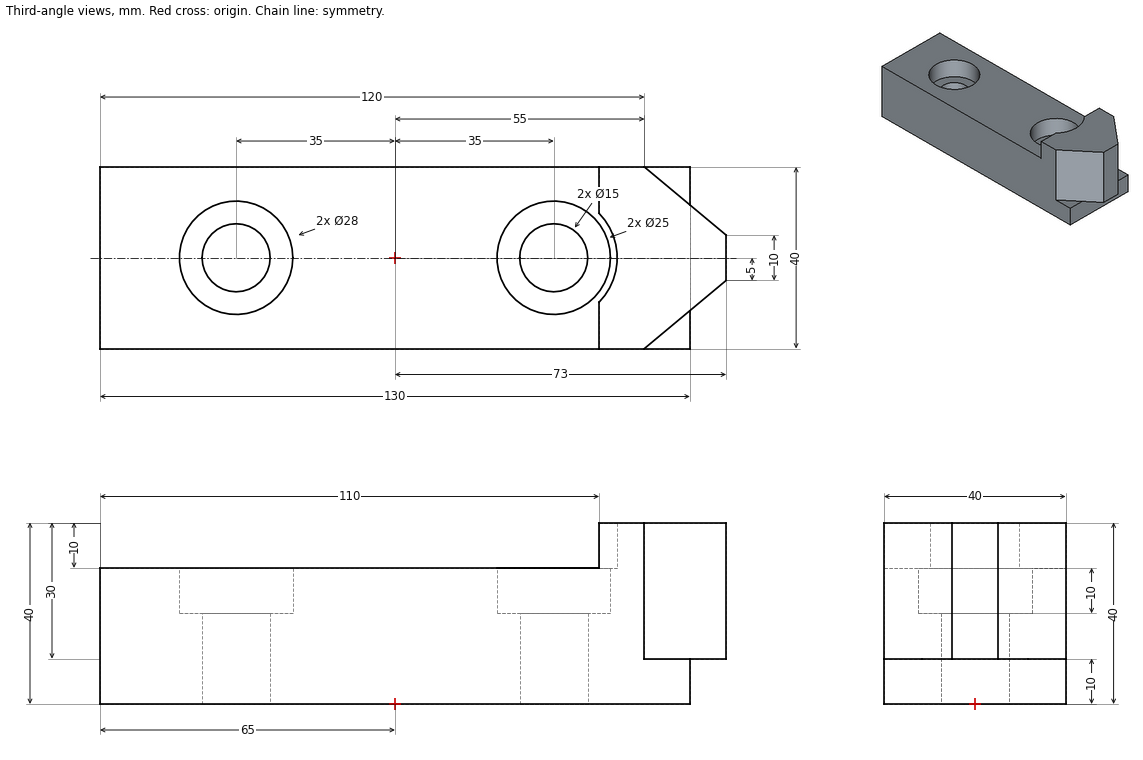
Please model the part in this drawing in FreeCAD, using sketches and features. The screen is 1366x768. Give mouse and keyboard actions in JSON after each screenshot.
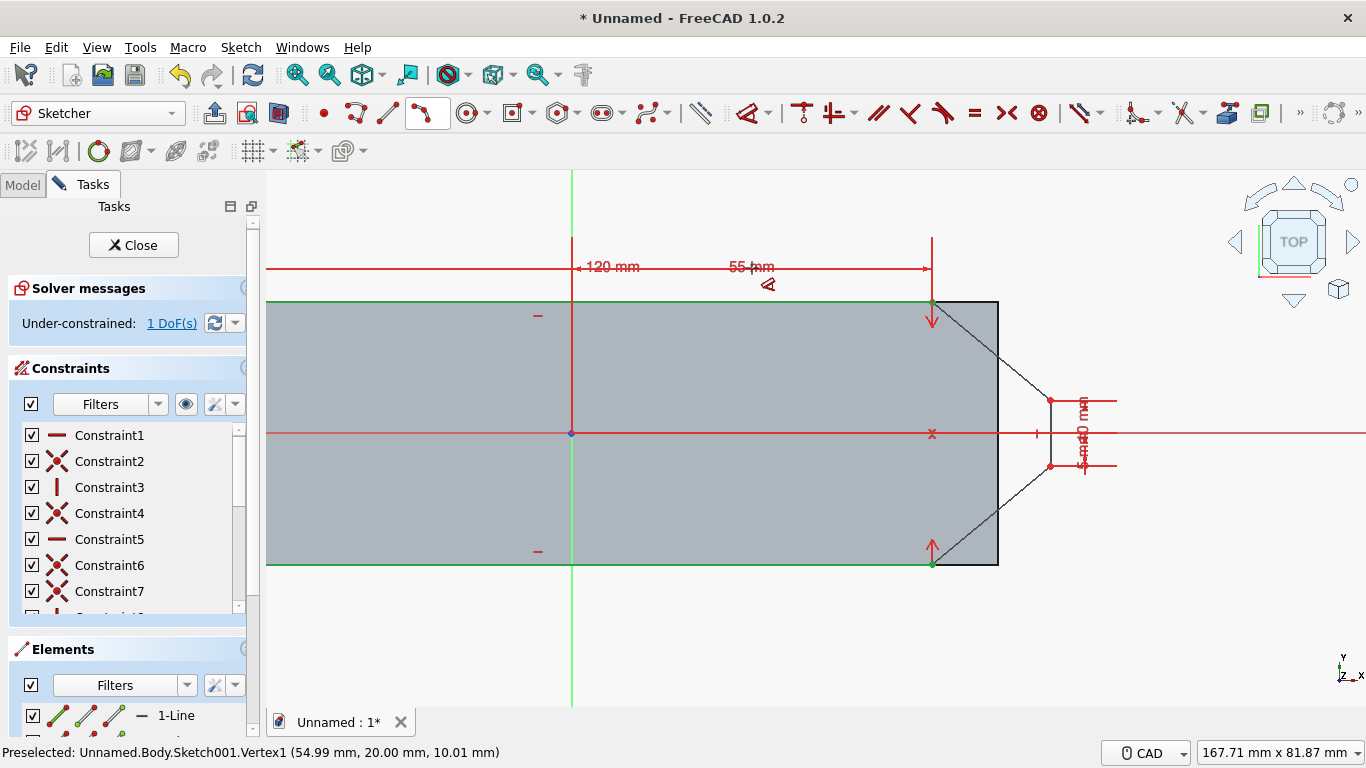
{"action": "left_click", "coordinate": [1051, 466]}
{"action": "left_click", "coordinate": [811, 500]}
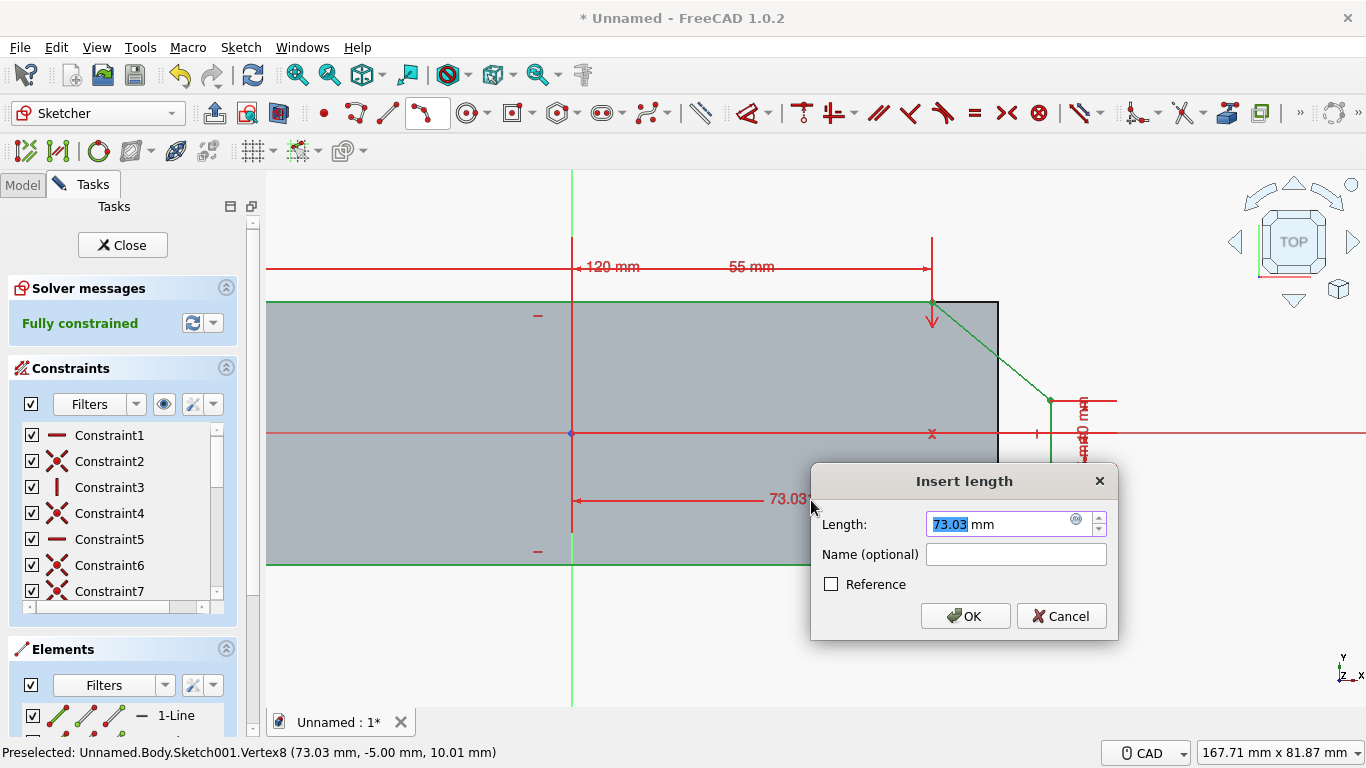
{"action": "type", "text": "73"}
{"action": "key", "text": "Return"}
{"action": "key", "text": "Escape"}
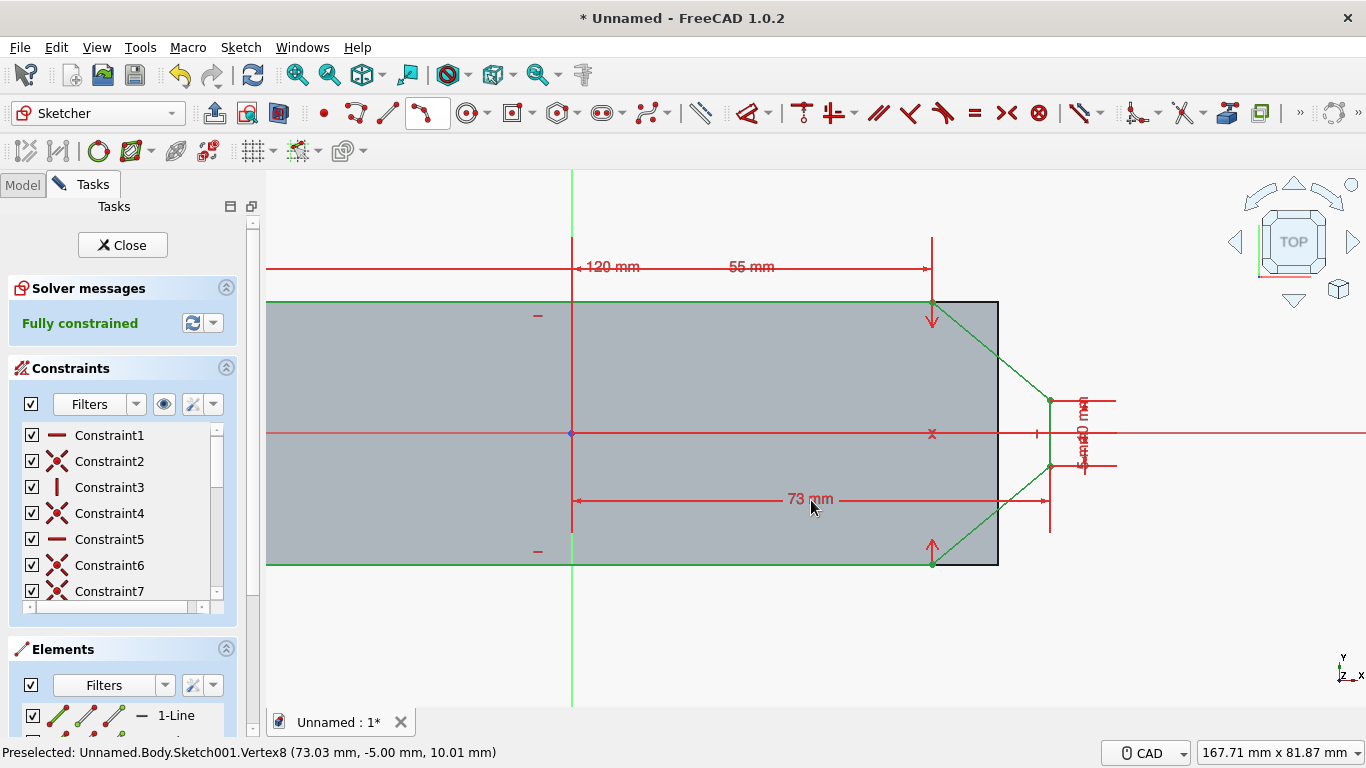
{"action": "left_click", "coordinate": [123, 245]}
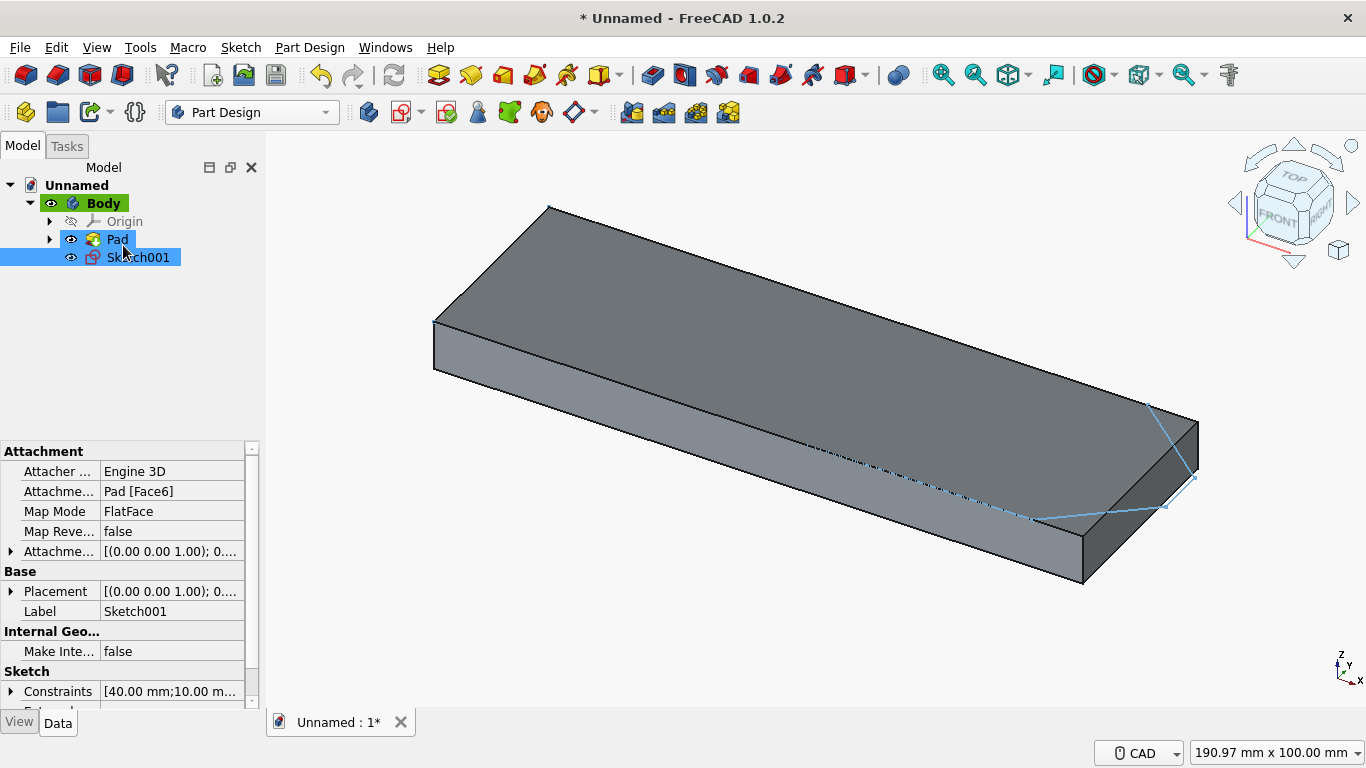
{"action": "left_click", "coordinate": [440, 76]}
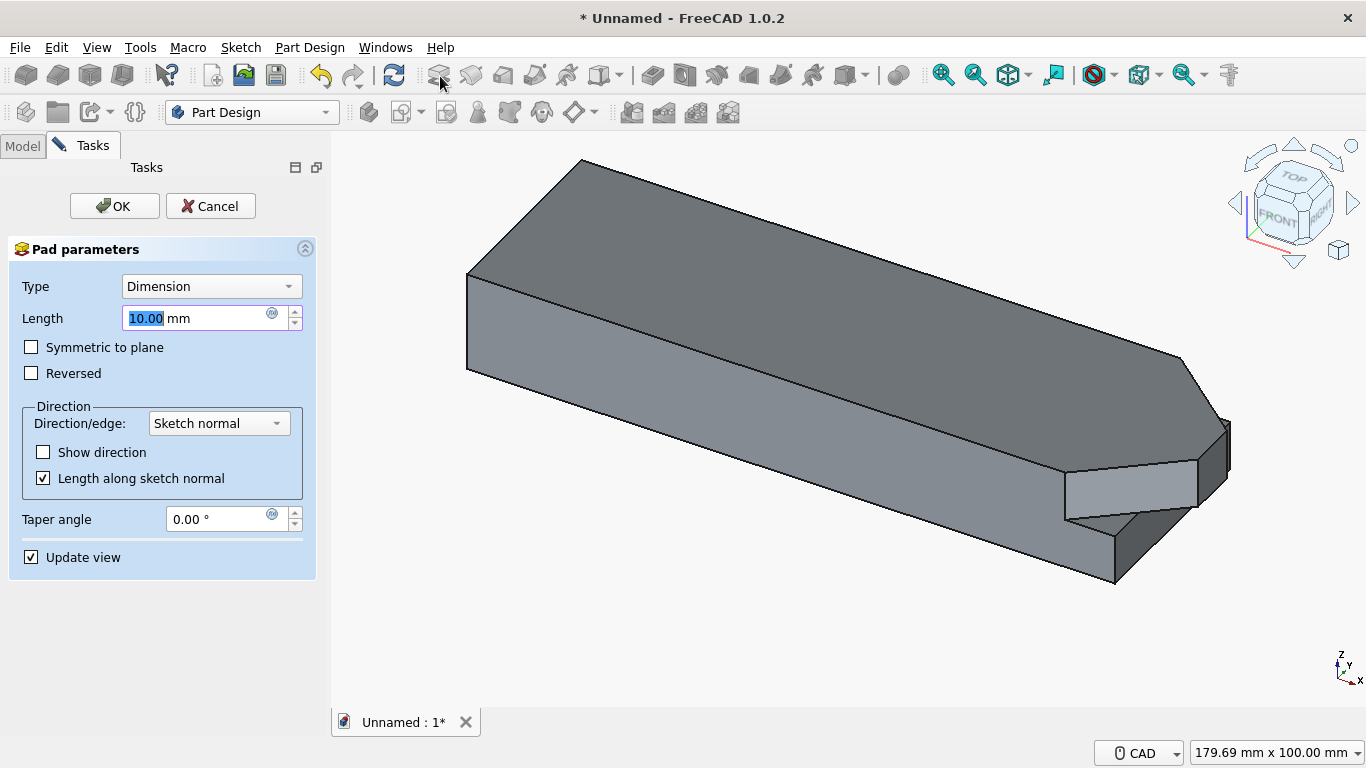
{"action": "type", "text": "30"}
{"action": "key", "text": "Tab"}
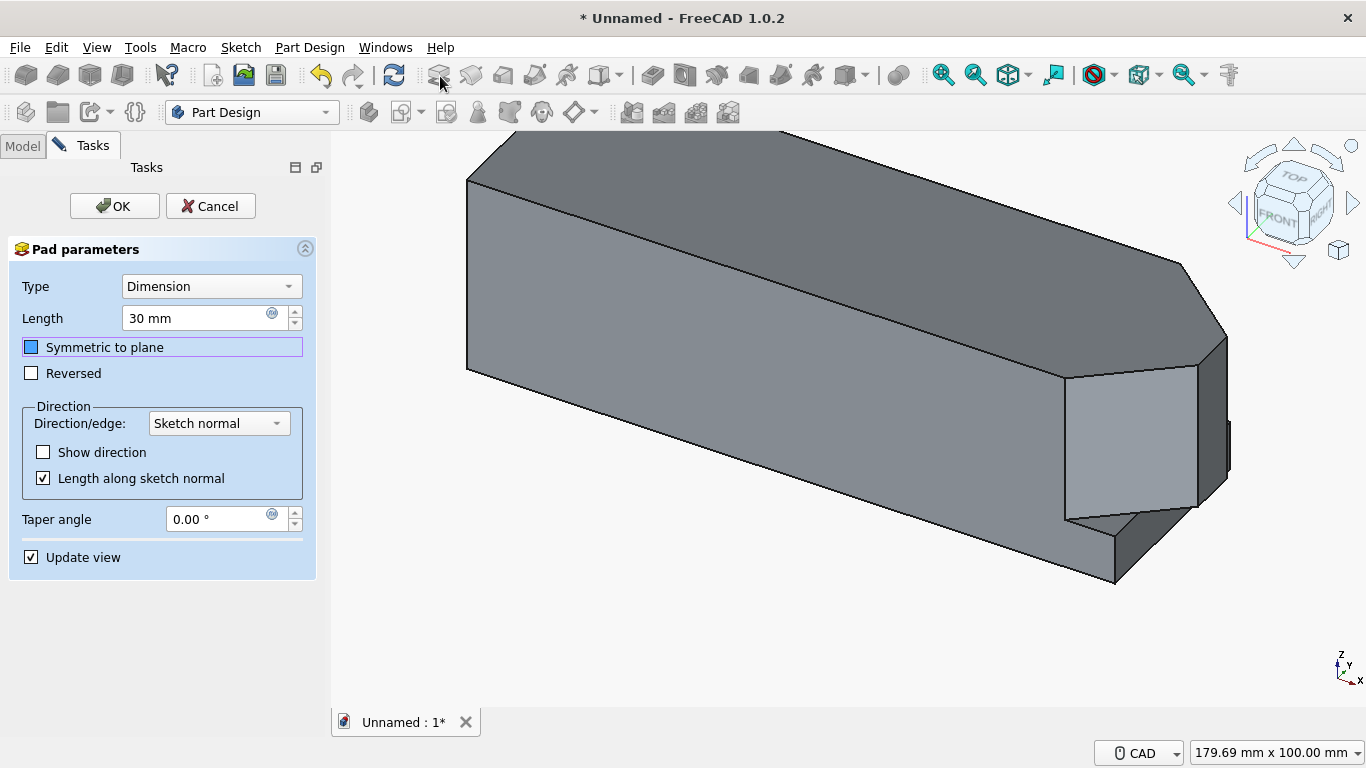
{"action": "left_click", "coordinate": [115, 206]}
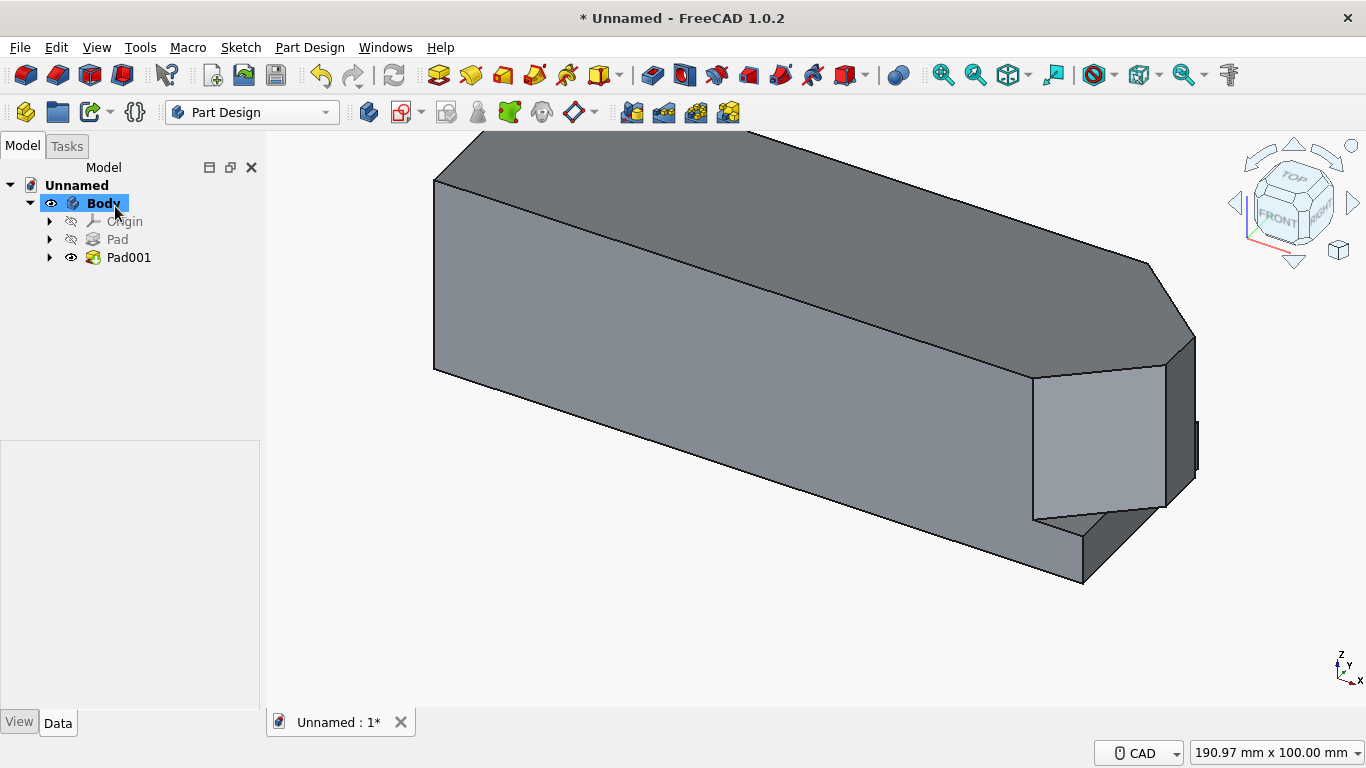
{"action": "key", "text": "v f"}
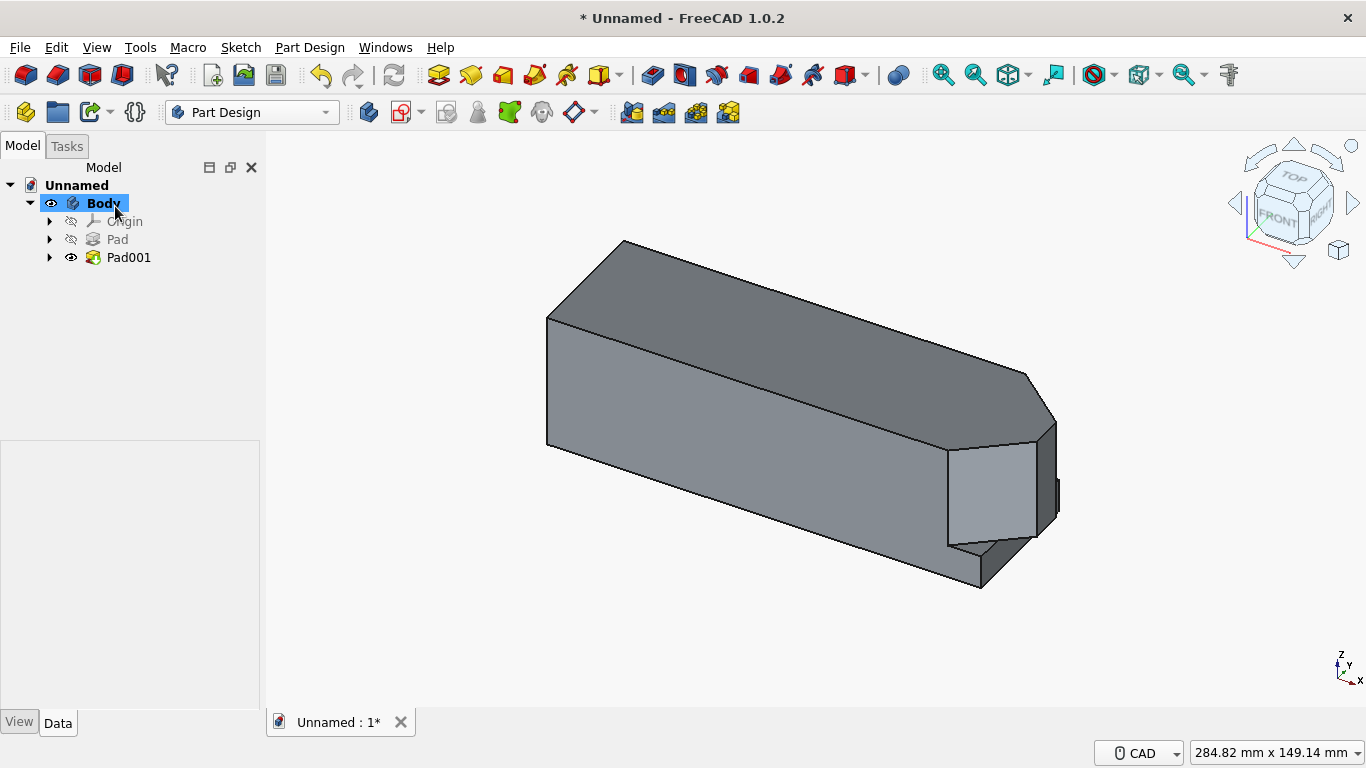
{"action": "left_click", "coordinate": [826, 473]}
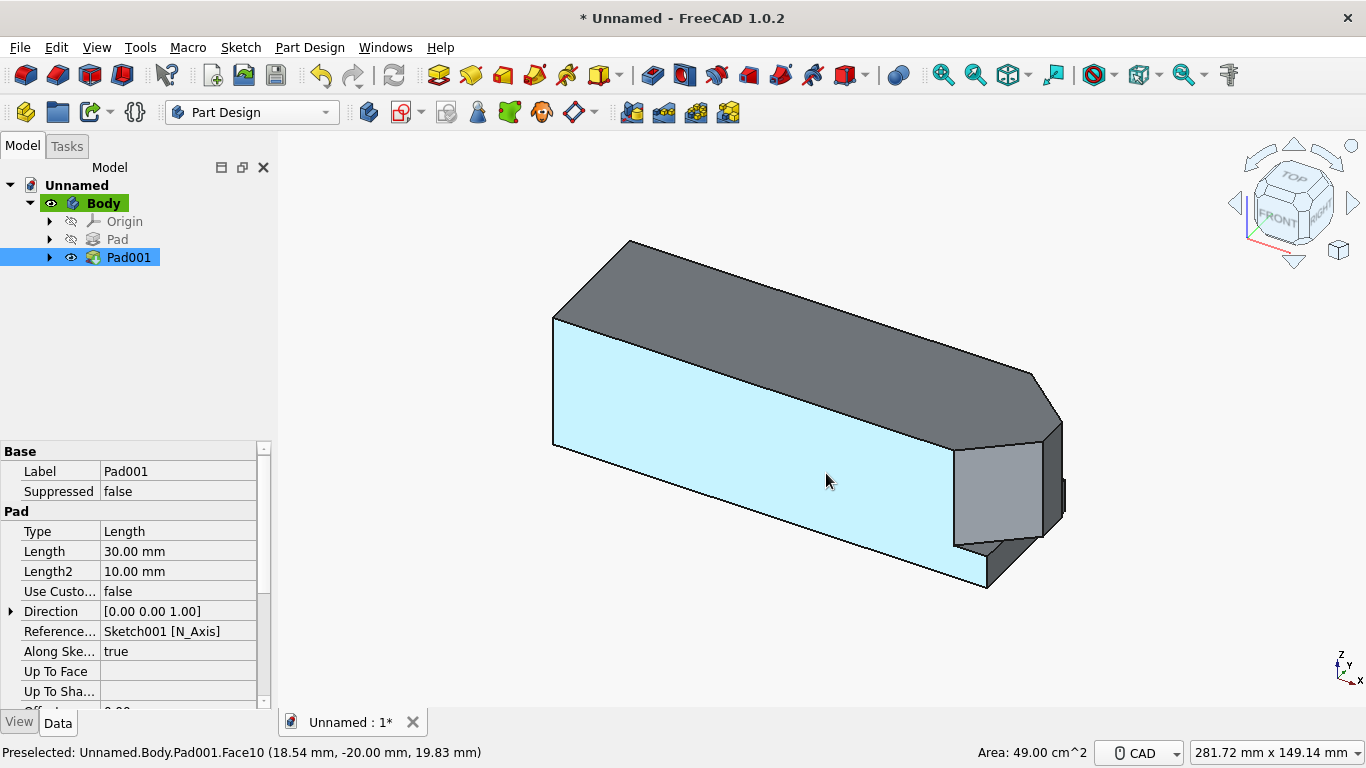
{"action": "left_click", "coordinate": [402, 112]}